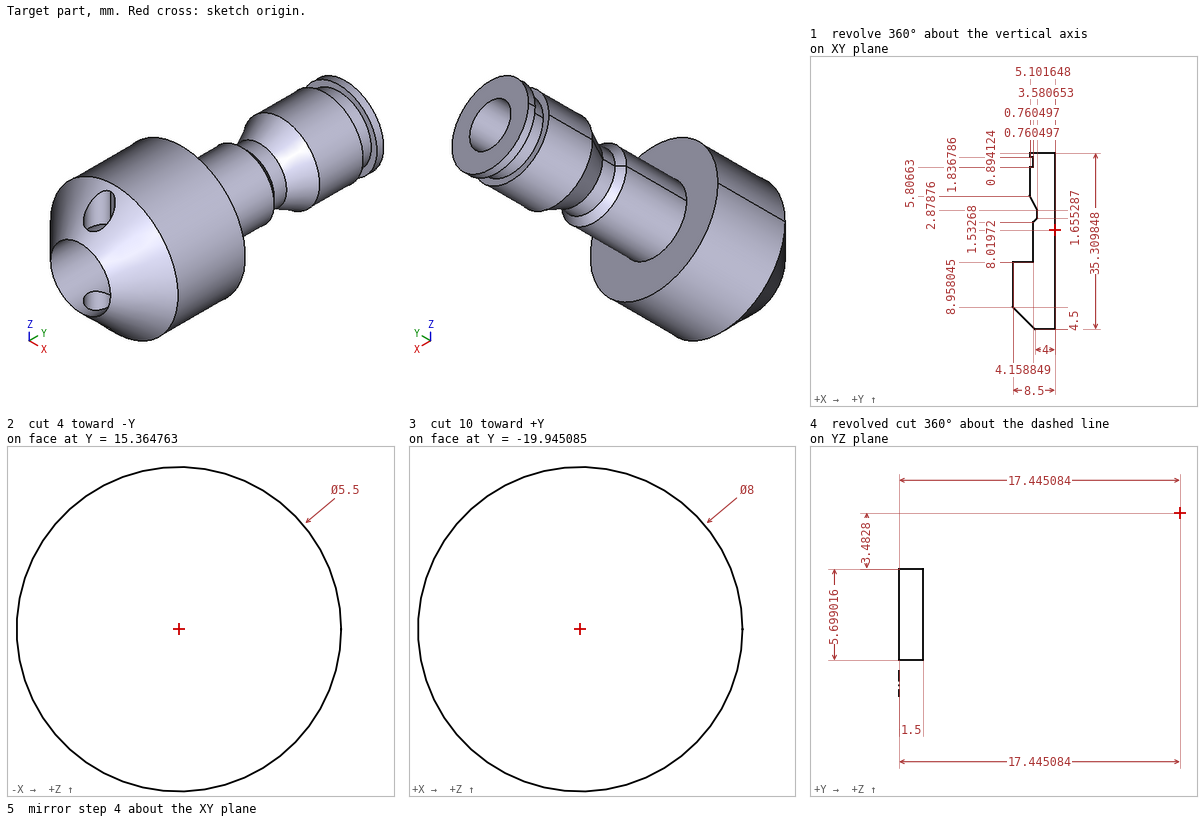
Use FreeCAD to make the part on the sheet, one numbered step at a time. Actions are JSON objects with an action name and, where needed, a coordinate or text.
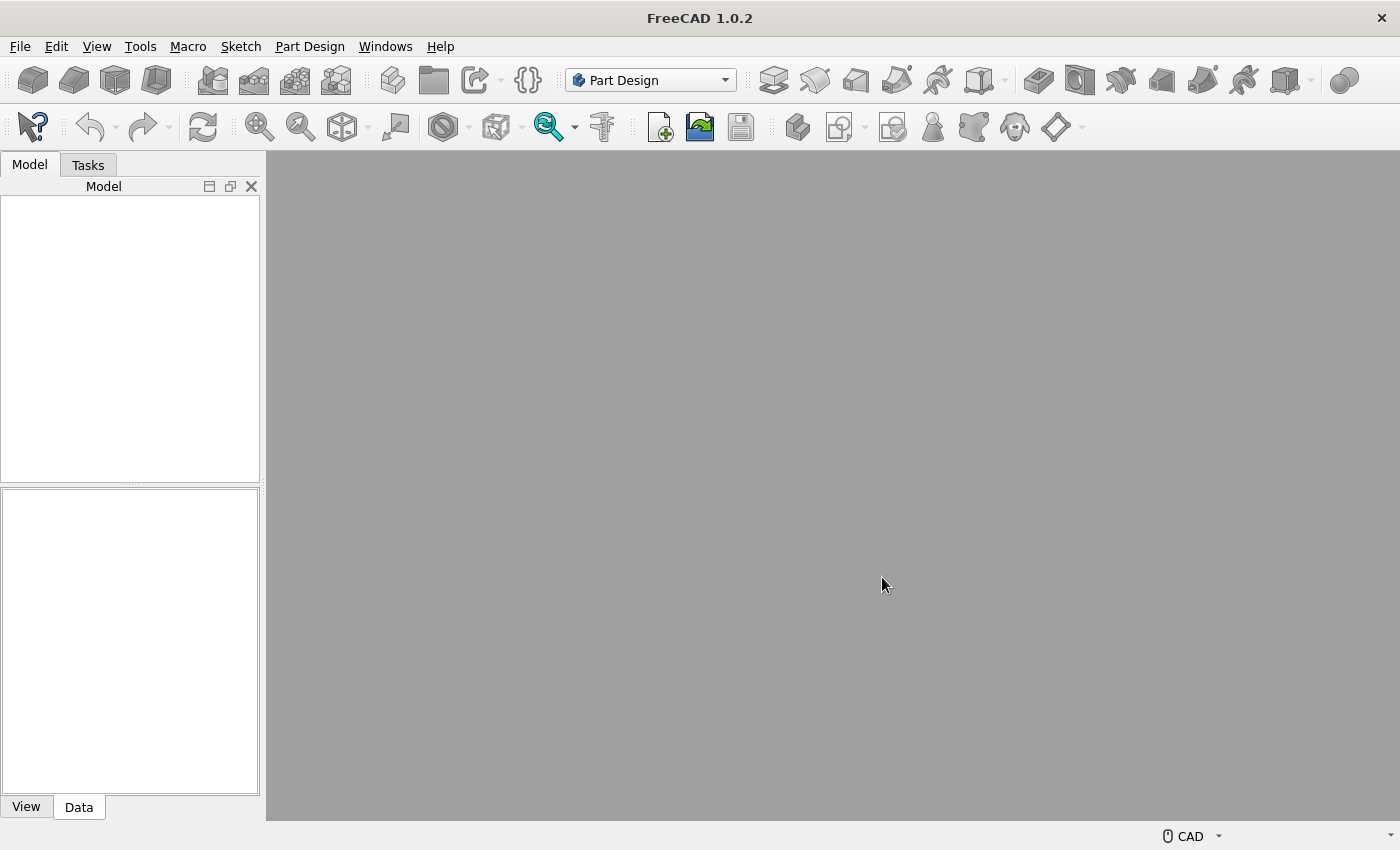
{"action": "left_click", "coordinate": [659, 128]}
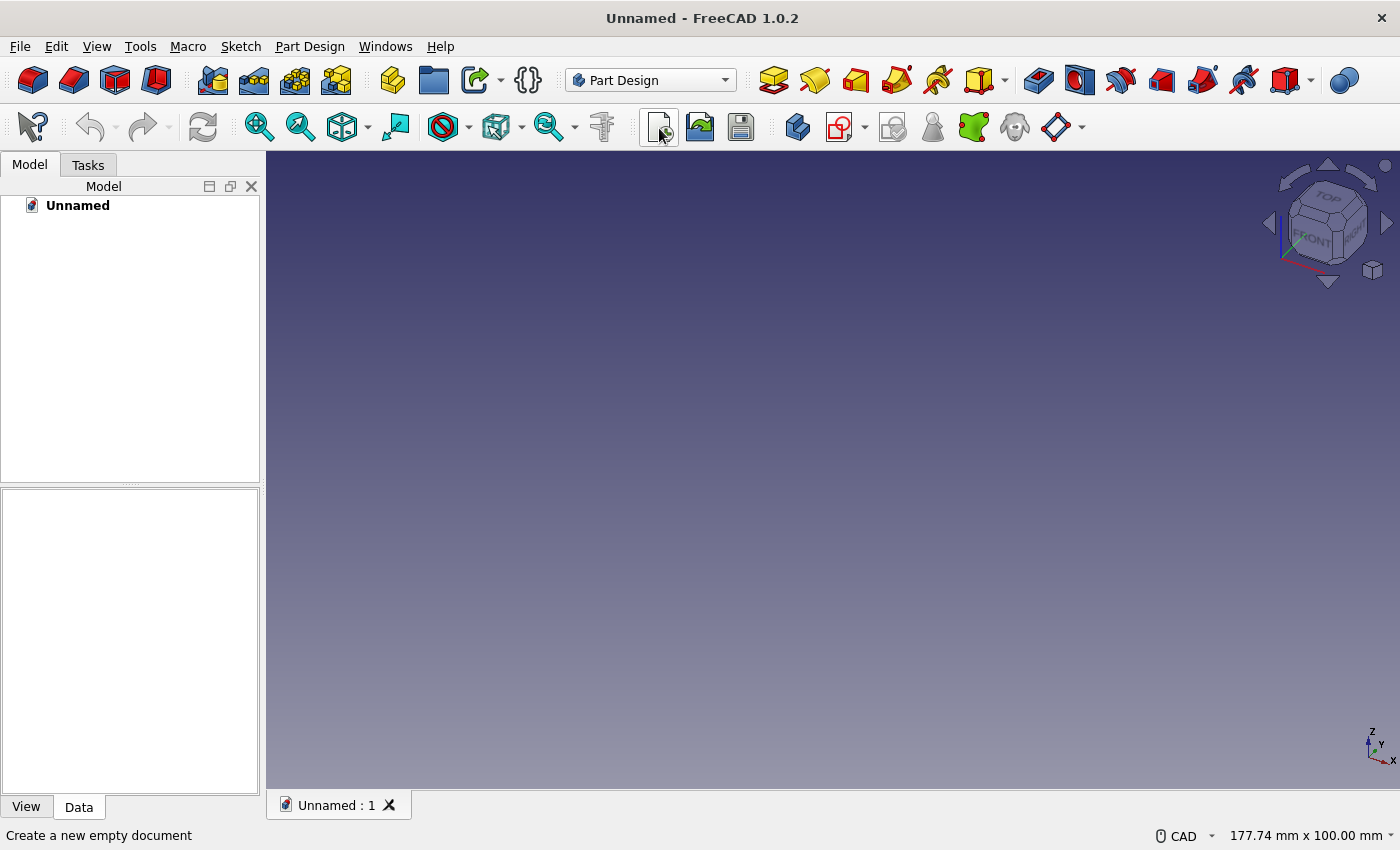
{"action": "left_click", "coordinate": [838, 128]}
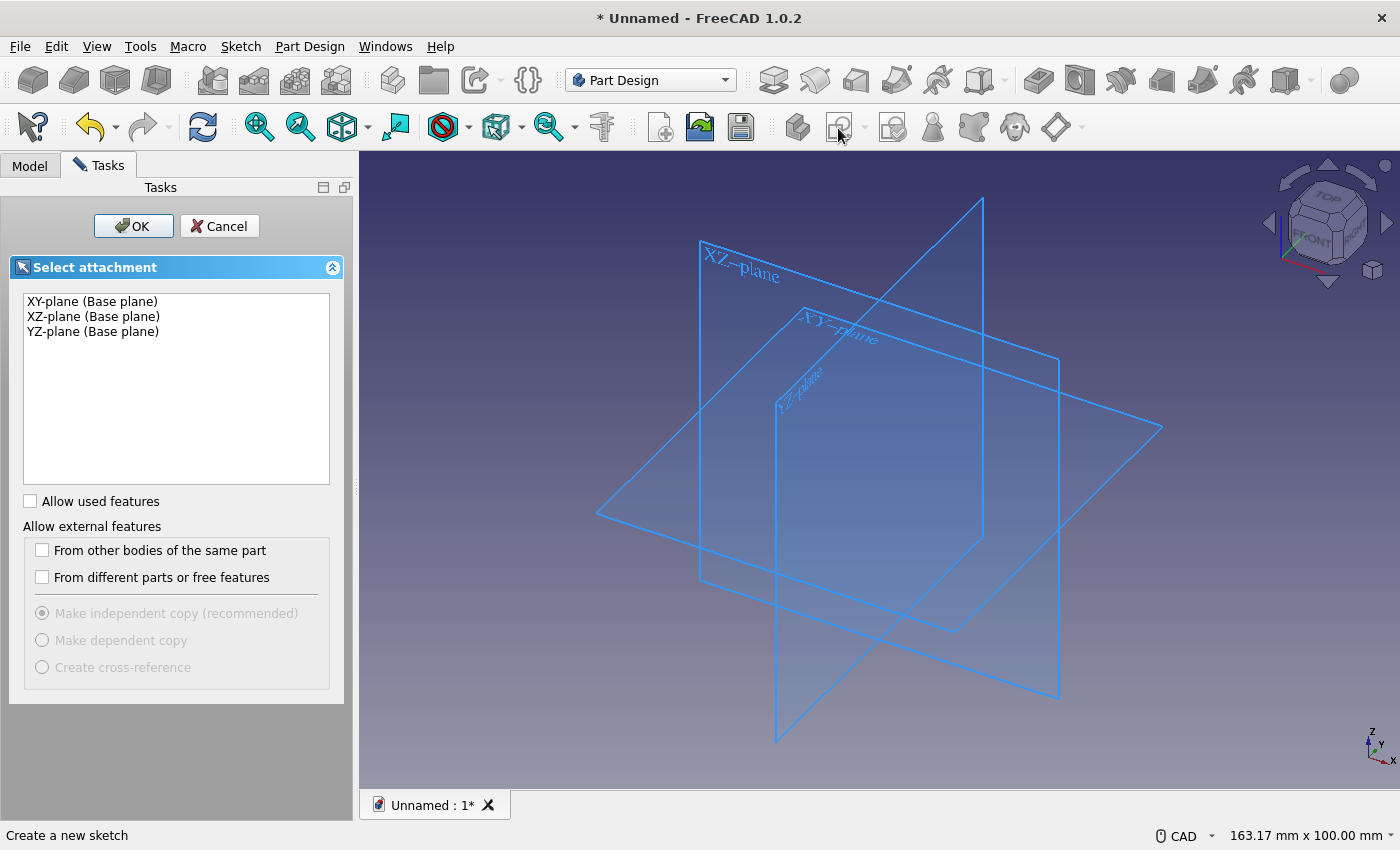
{"action": "left_click", "coordinate": [84, 302]}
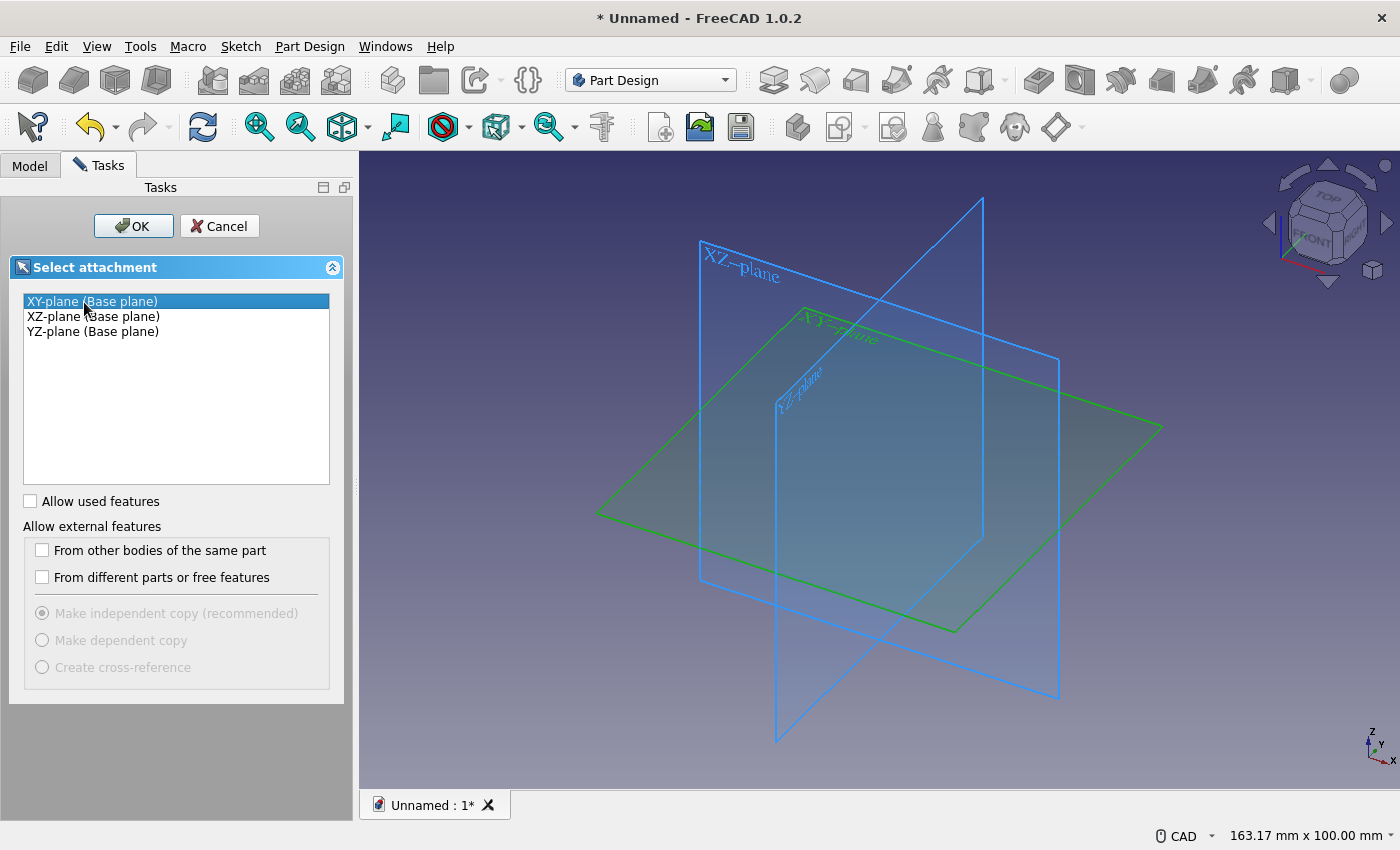
{"action": "left_click", "coordinate": [134, 226]}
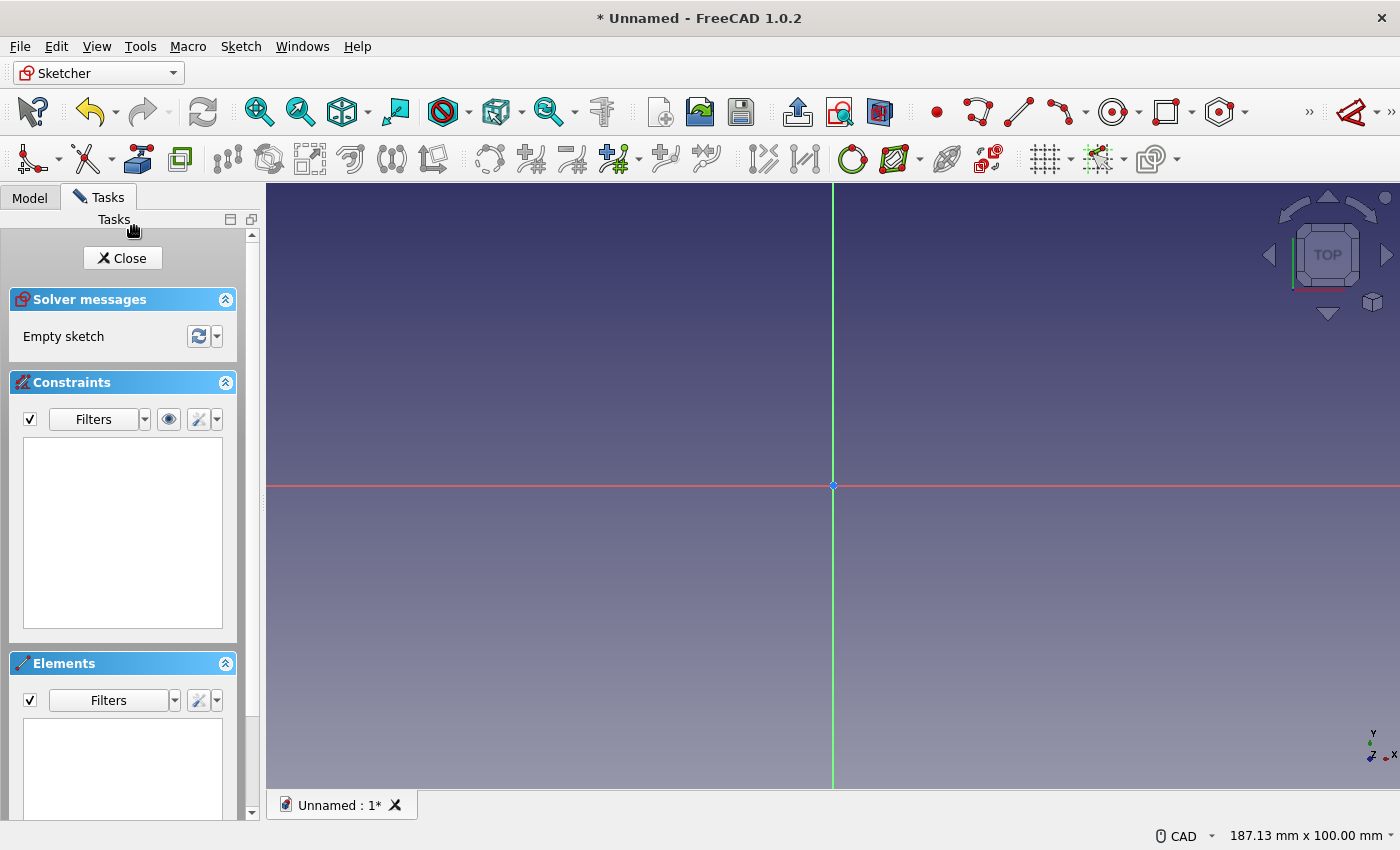
{"action": "scroll", "coordinate": [859, 517], "scroll_direction": "up", "scroll_amount": 3}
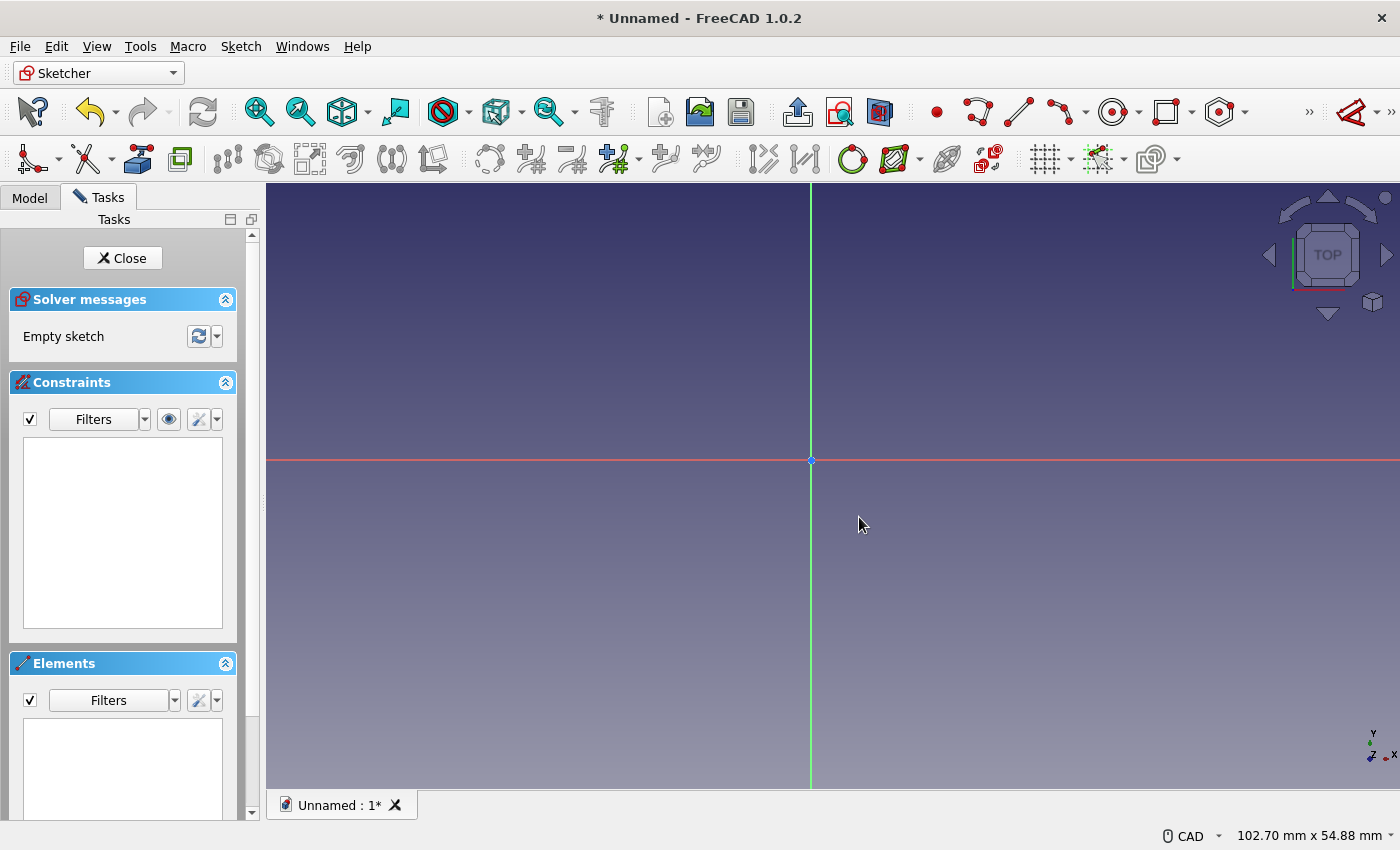
{"action": "left_click", "coordinate": [978, 112]}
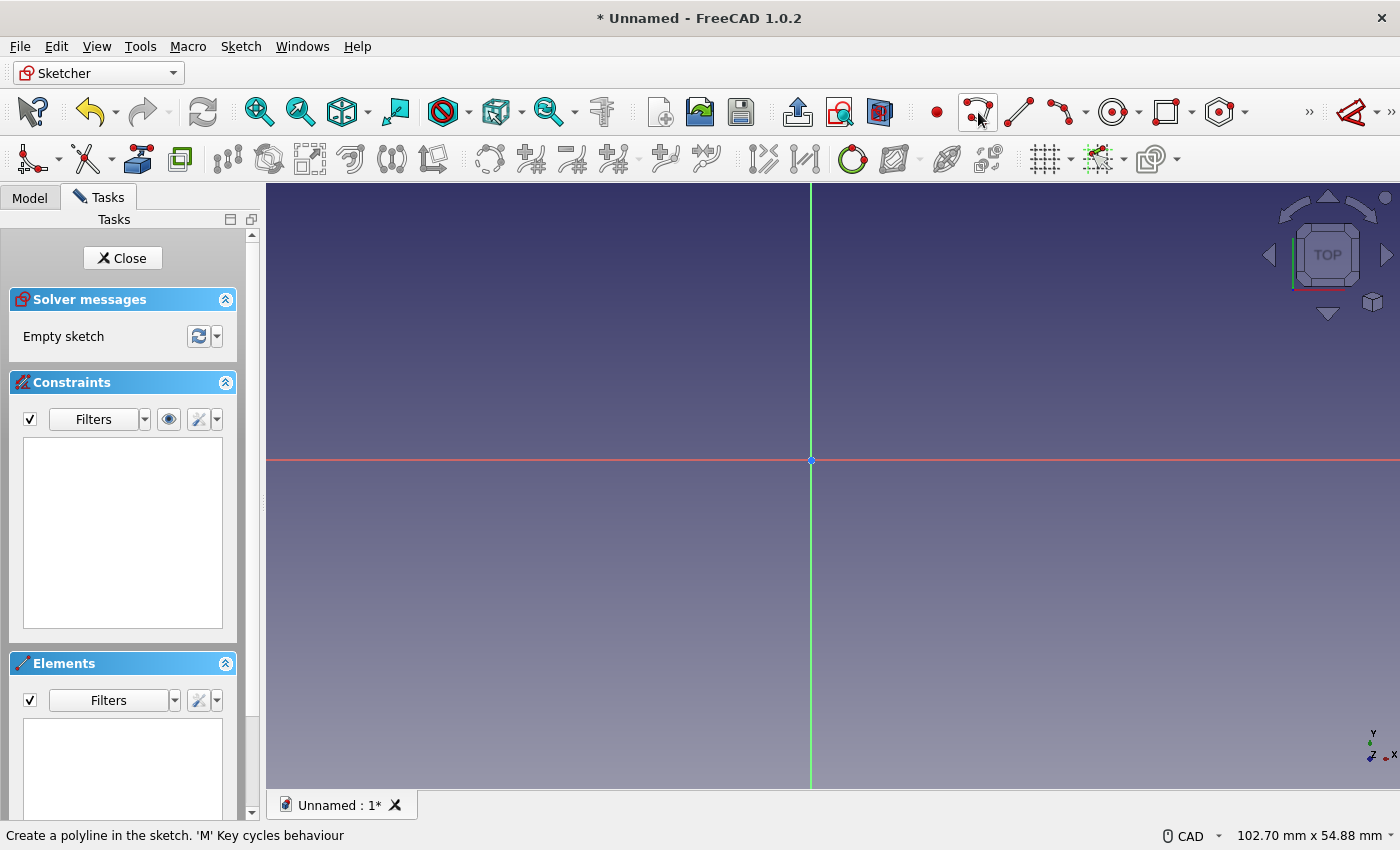
{"action": "left_click", "coordinate": [772, 435]}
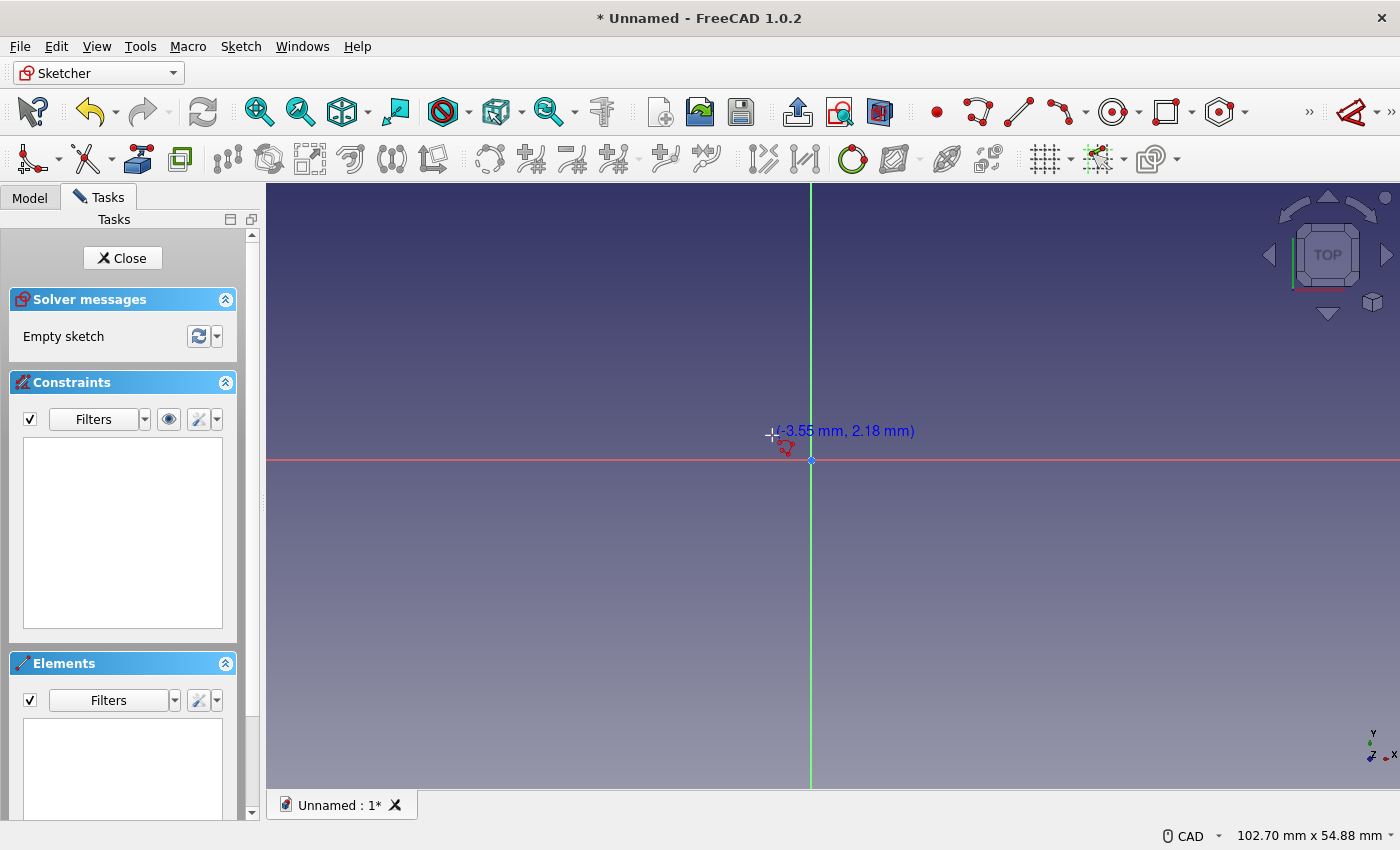
{"action": "scroll", "coordinate": [763, 443], "scroll_direction": "up", "scroll_amount": 2}